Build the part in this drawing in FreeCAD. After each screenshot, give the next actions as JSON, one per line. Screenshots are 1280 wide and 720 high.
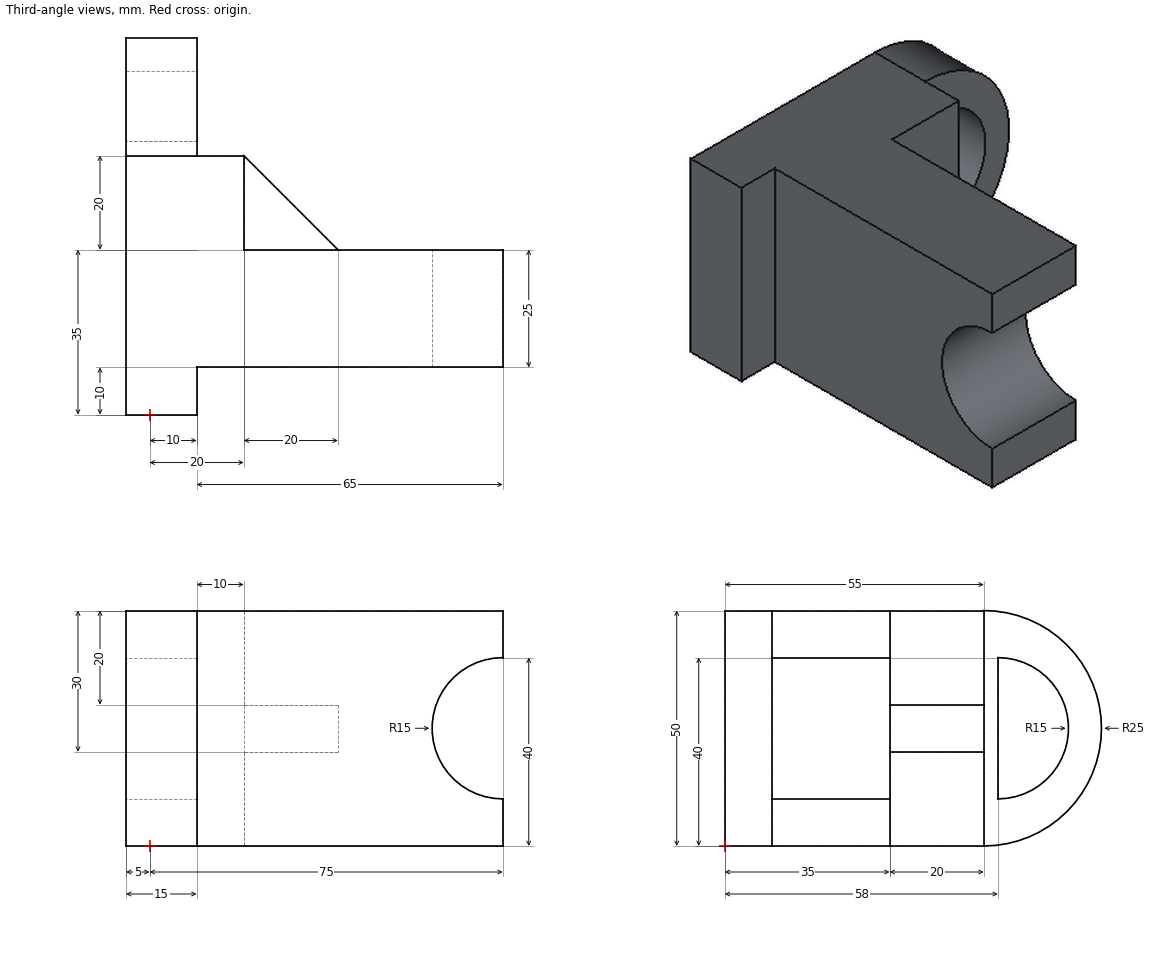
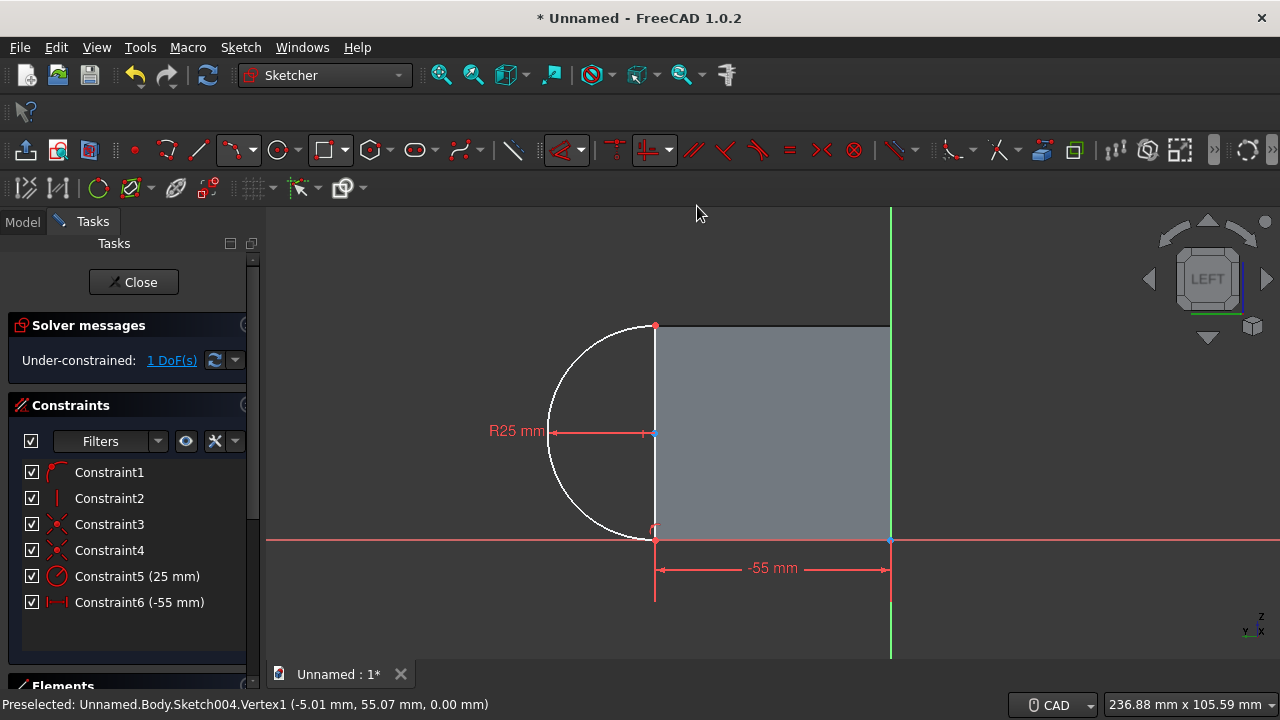
{"action": "left_click", "coordinate": [655, 433]}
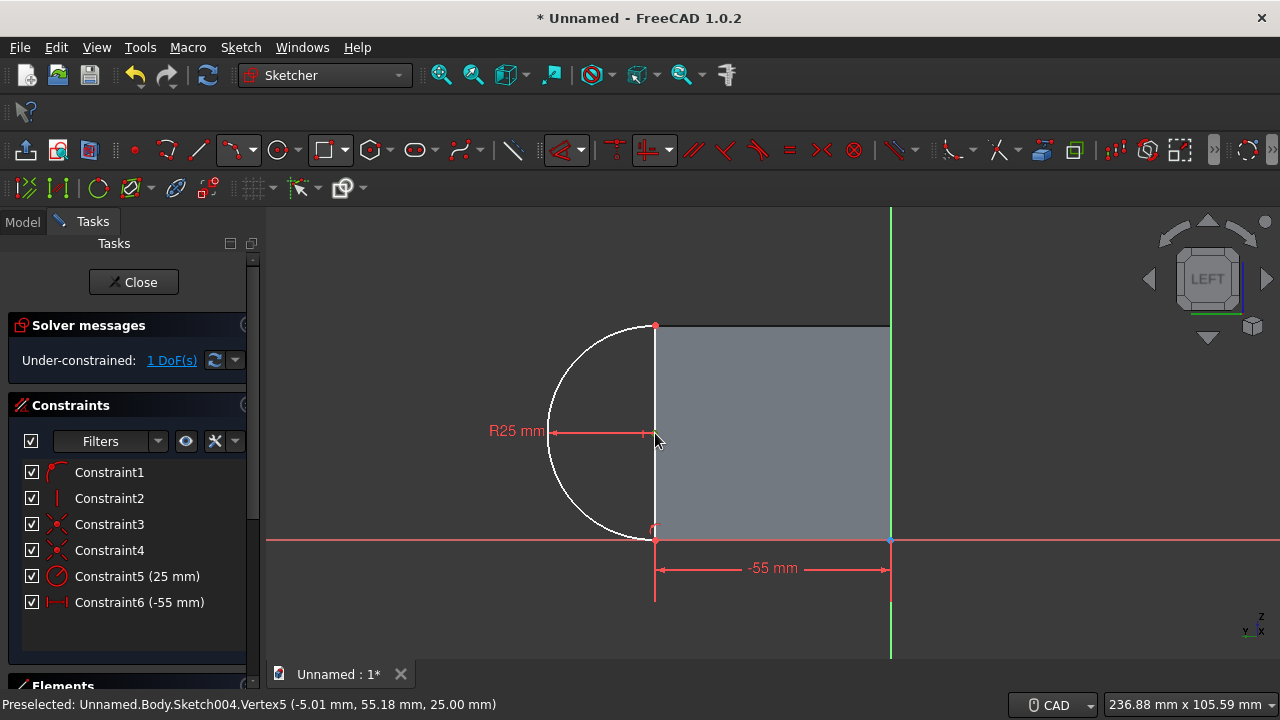
{"action": "key", "text": "l"}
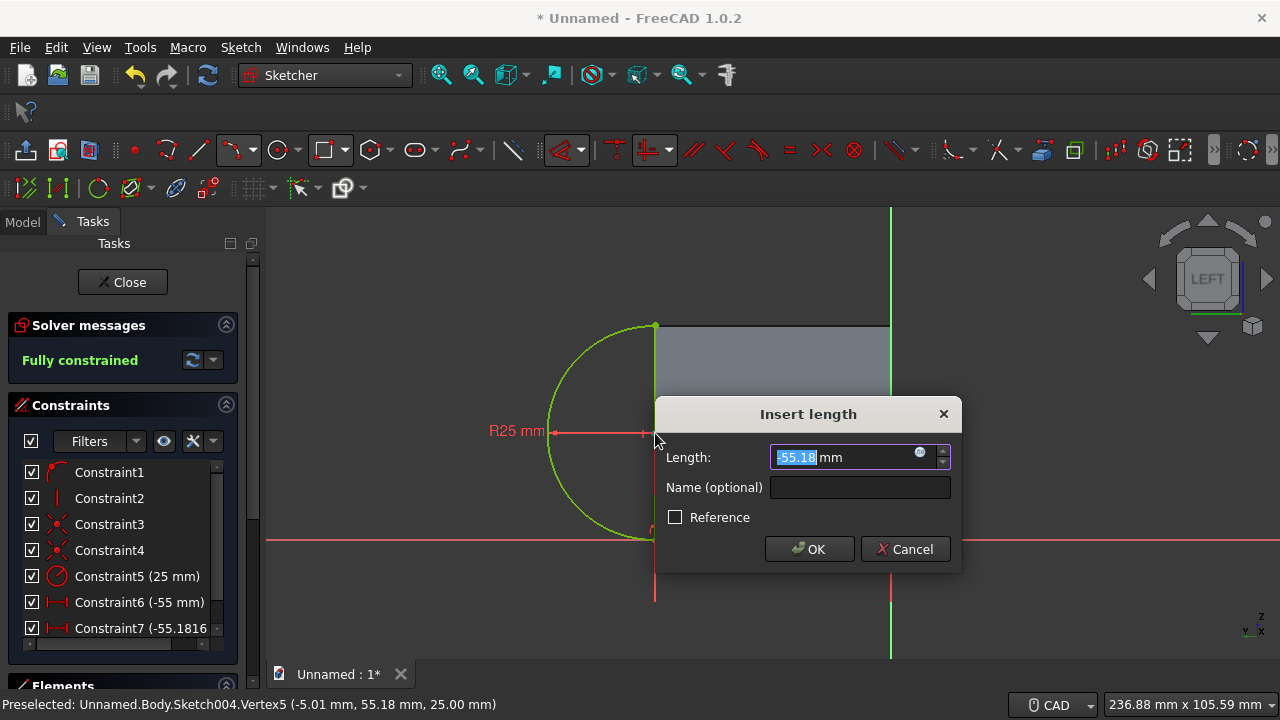
{"action": "type", "text": "-55"}
{"action": "key", "text": "Return"}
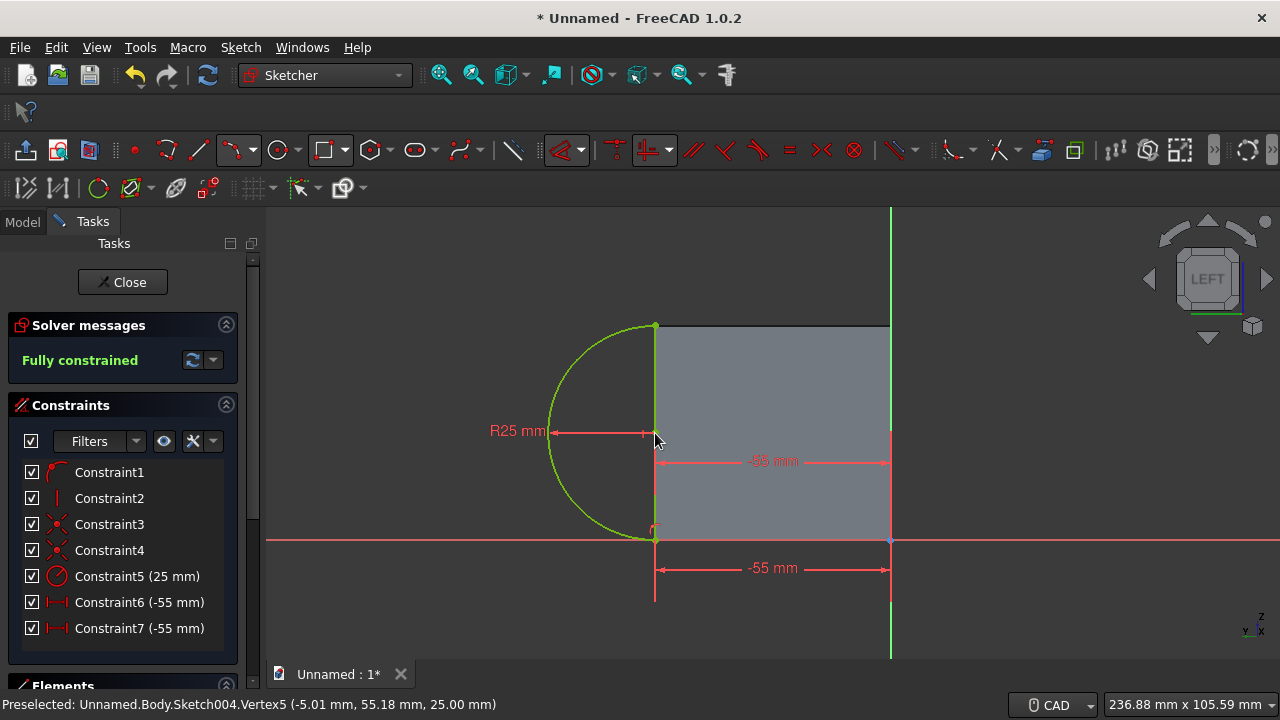
{"action": "left_click", "coordinate": [123, 282]}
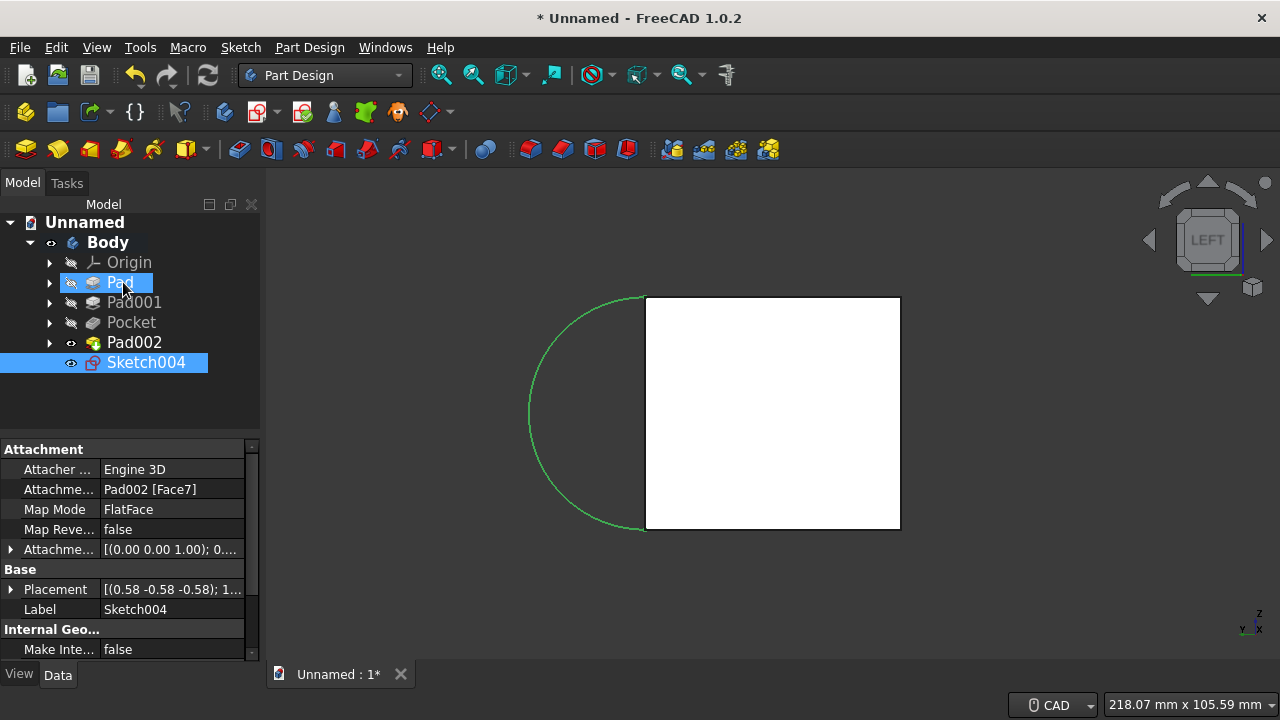
{"action": "left_click", "coordinate": [26, 150]}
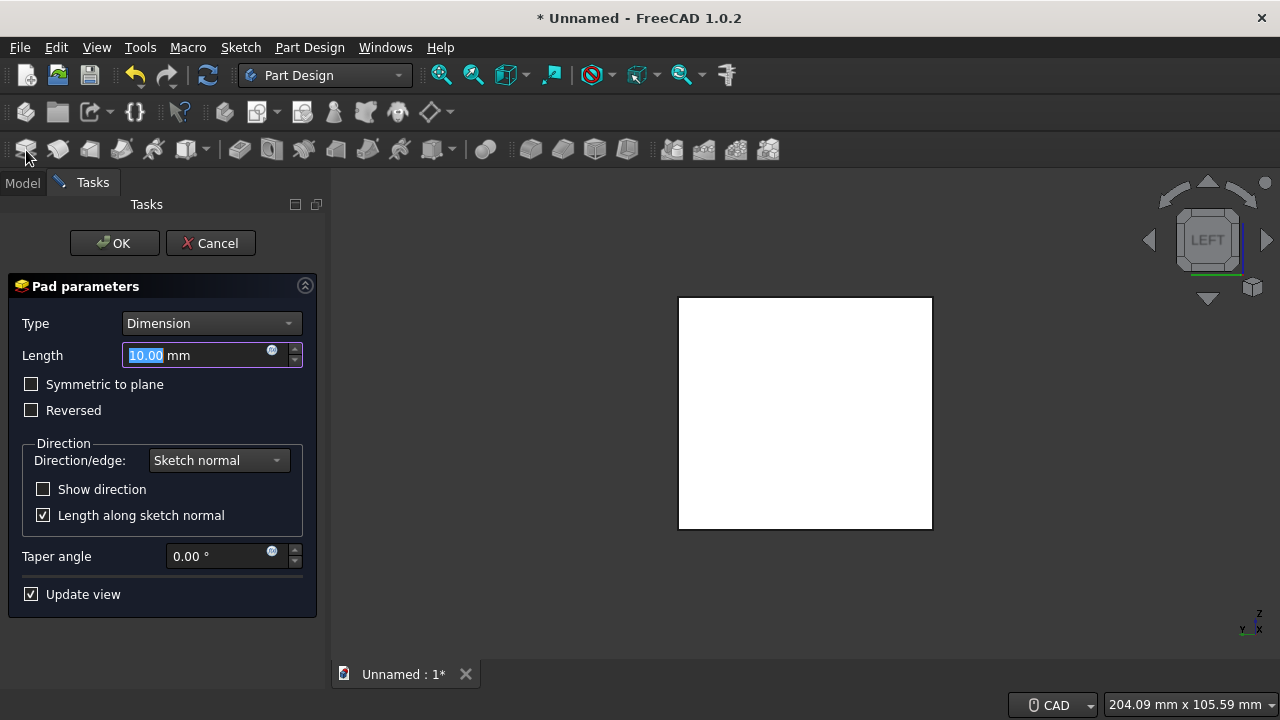
{"action": "type", "text": "15"}
{"action": "key", "text": "Tab"}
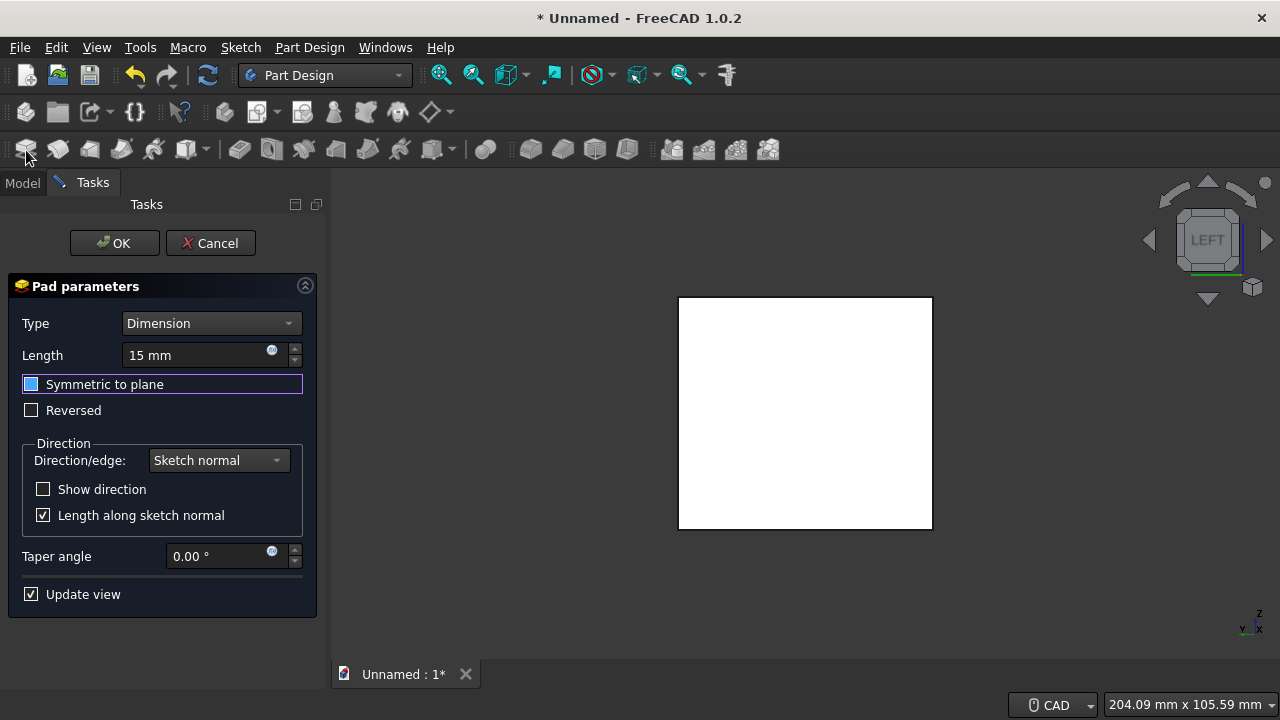
{"action": "left_click", "coordinate": [30, 410]}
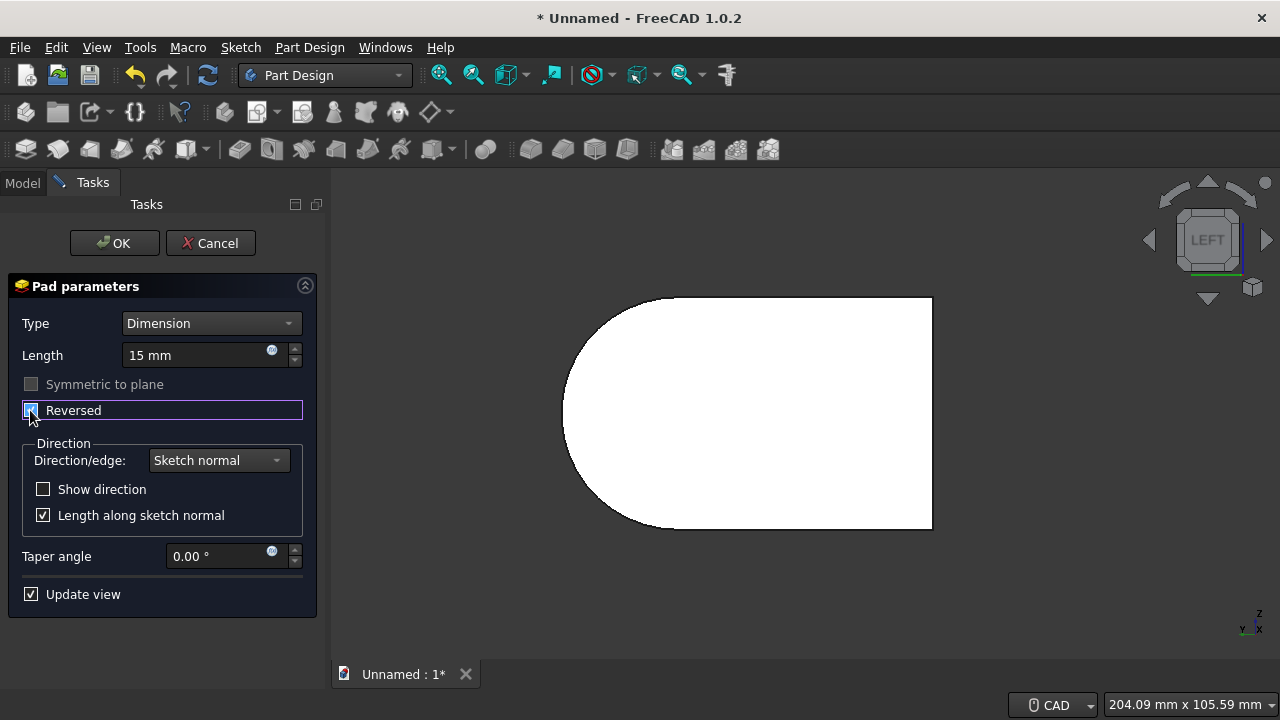
{"action": "left_click", "coordinate": [115, 243]}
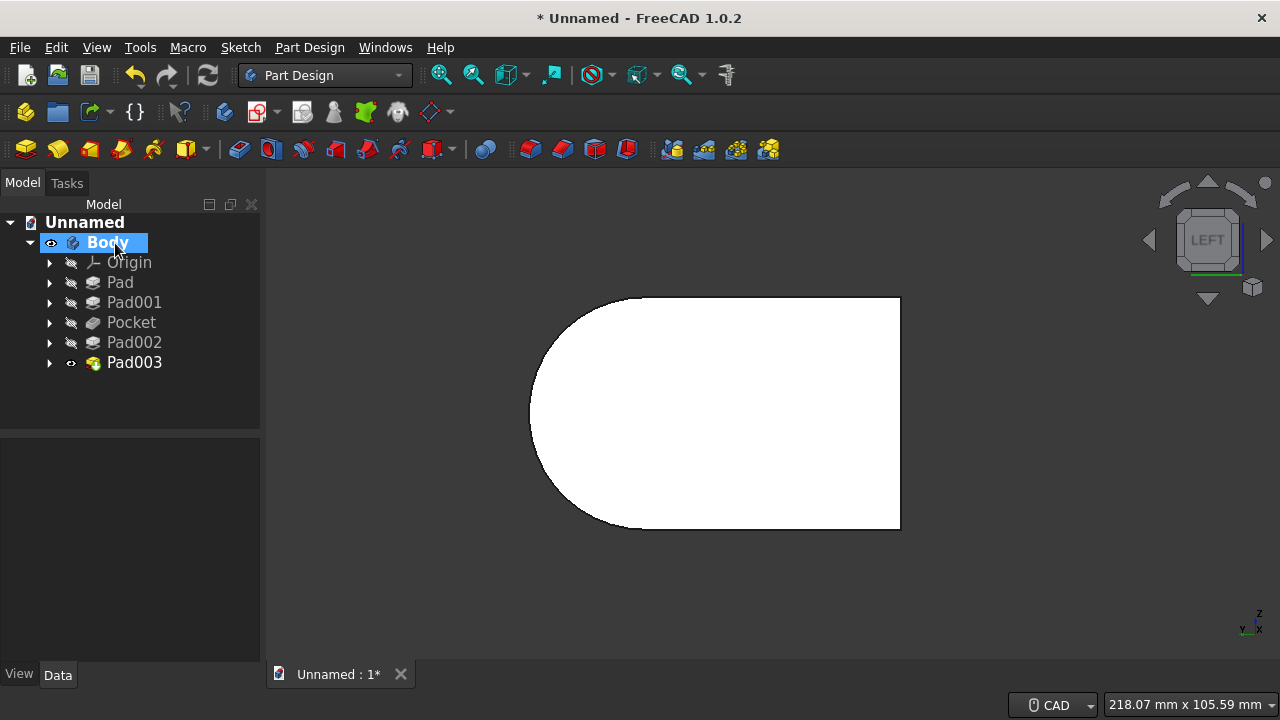
{"action": "key", "text": "0"}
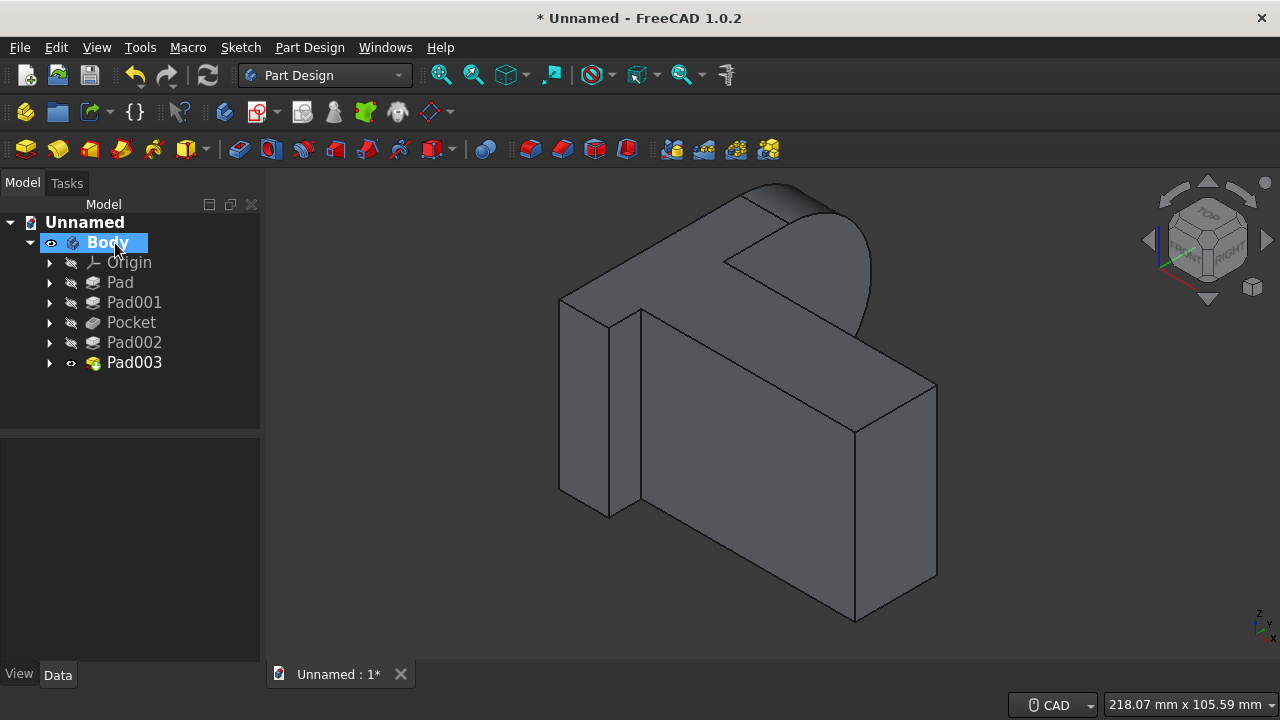
{"action": "left_click", "coordinate": [442, 76]}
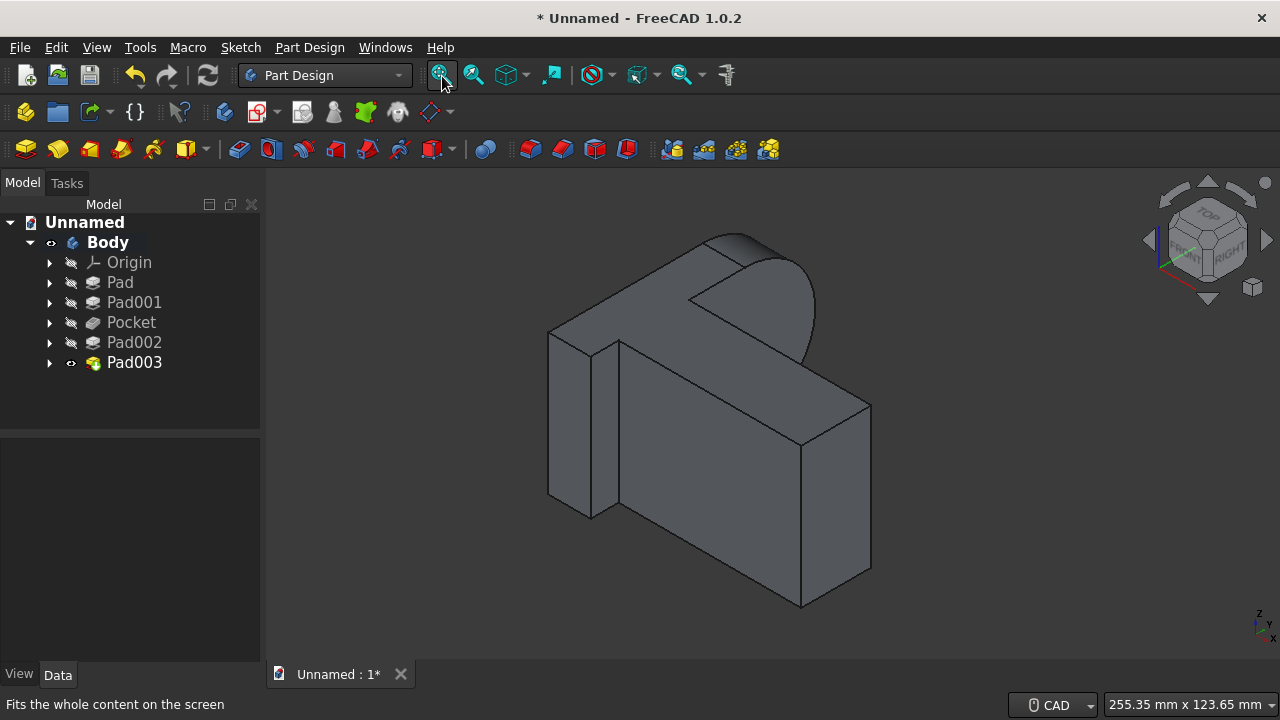
{"action": "left_click", "coordinate": [752, 320]}